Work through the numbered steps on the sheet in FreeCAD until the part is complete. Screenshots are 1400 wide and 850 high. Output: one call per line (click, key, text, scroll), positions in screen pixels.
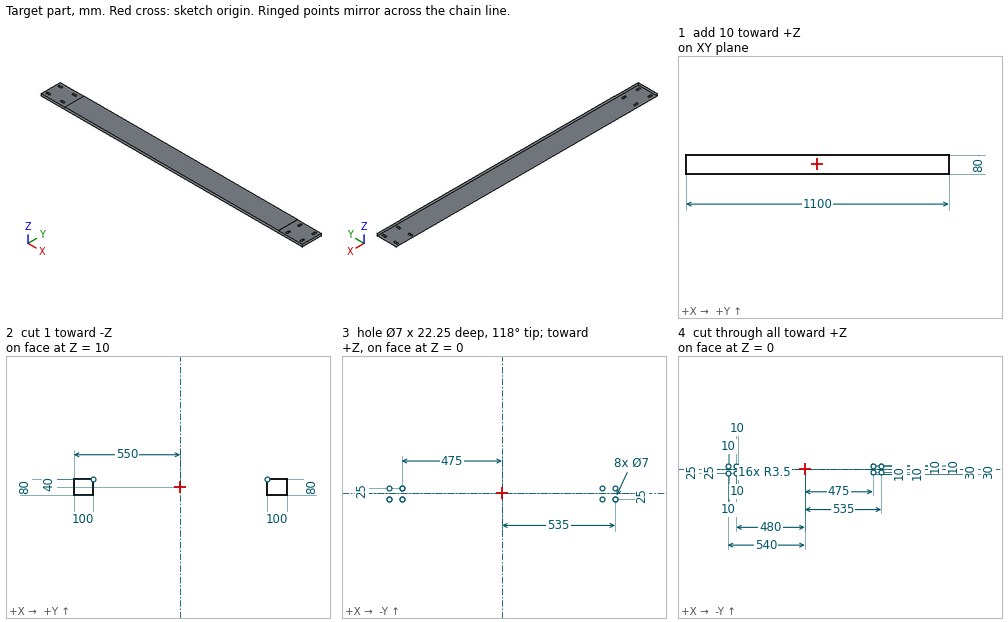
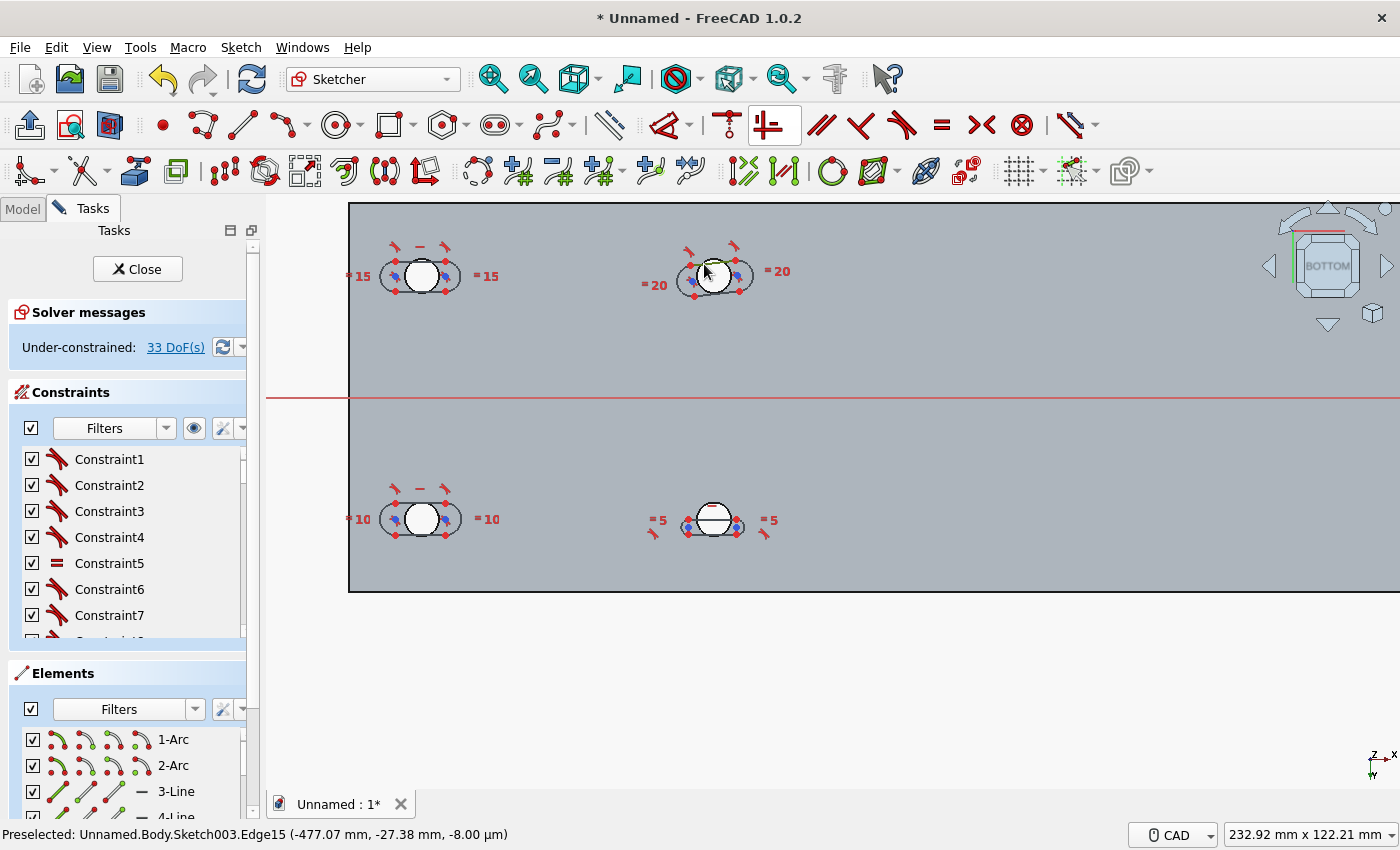
click(796, 126)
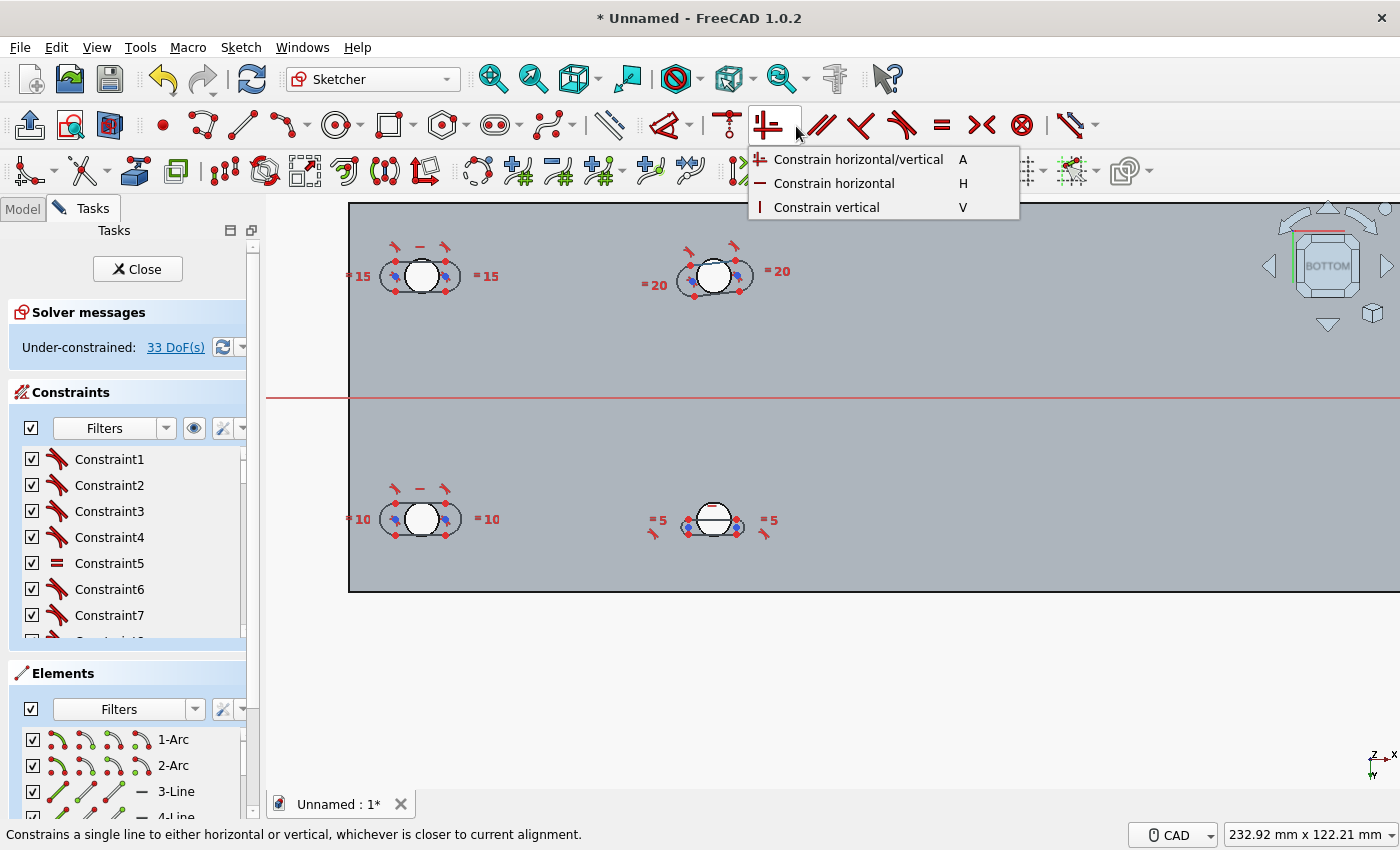
click(884, 183)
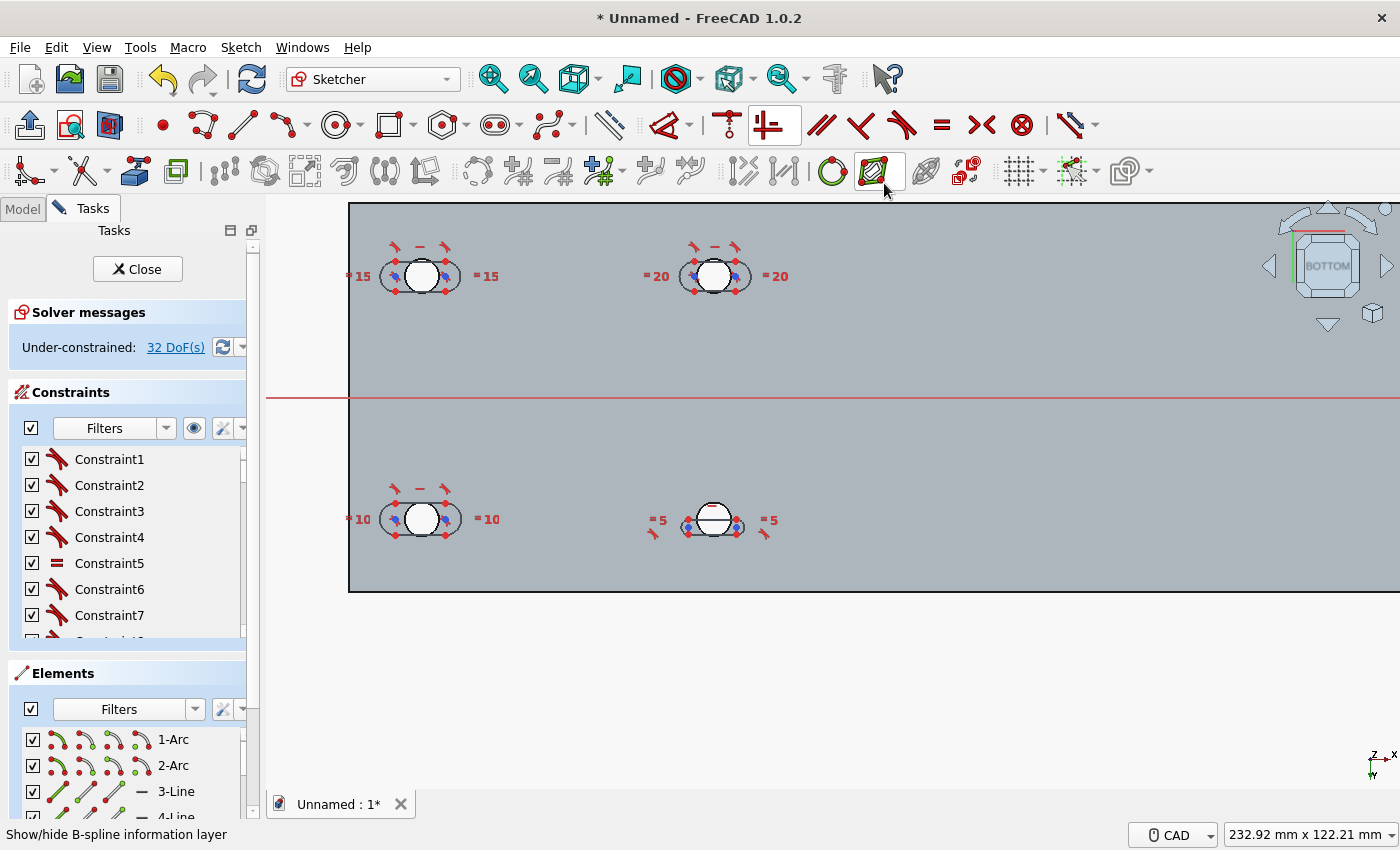
scroll(681, 527, up, 3)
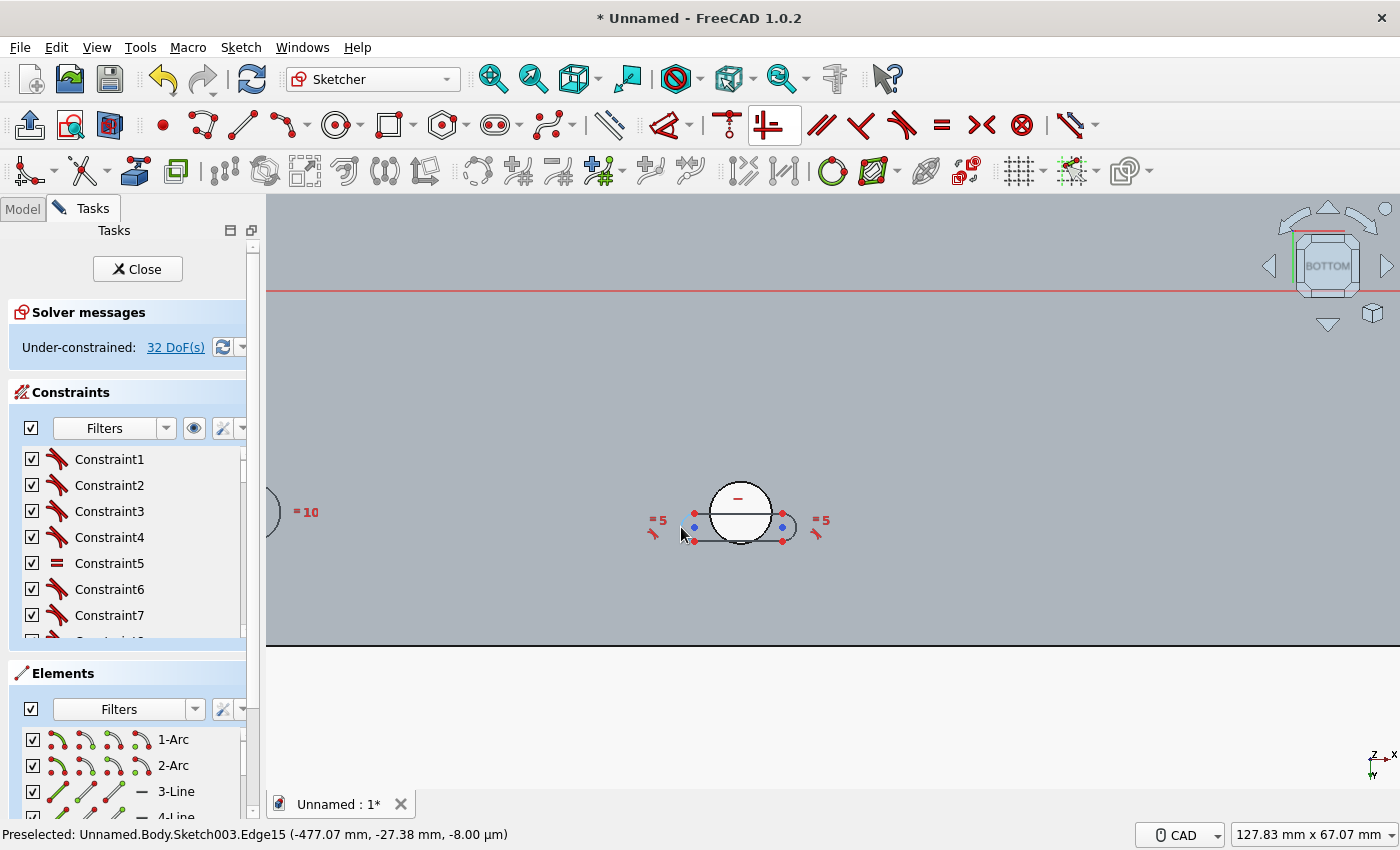
click(681, 527)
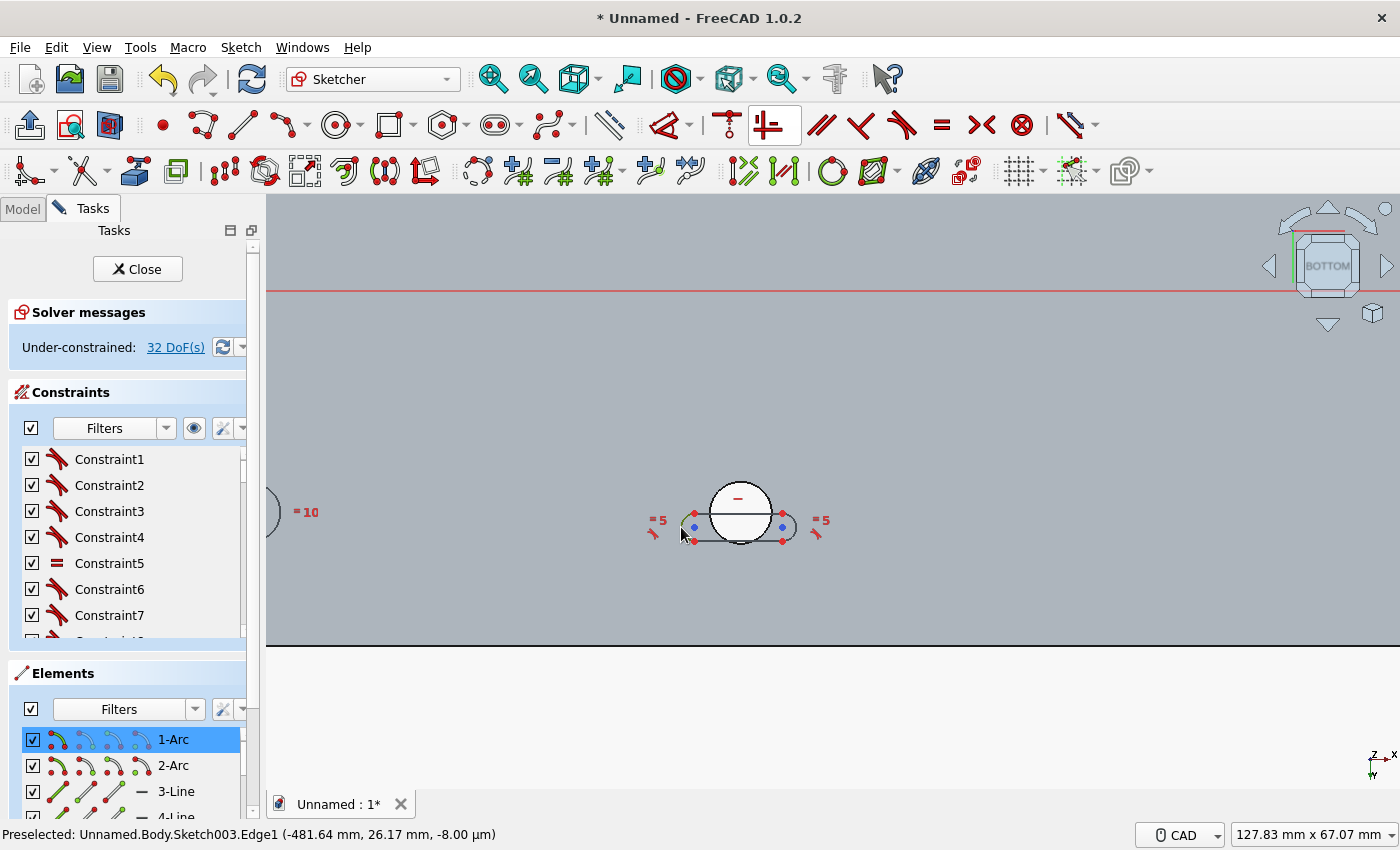
scroll(430, 508, down, 13)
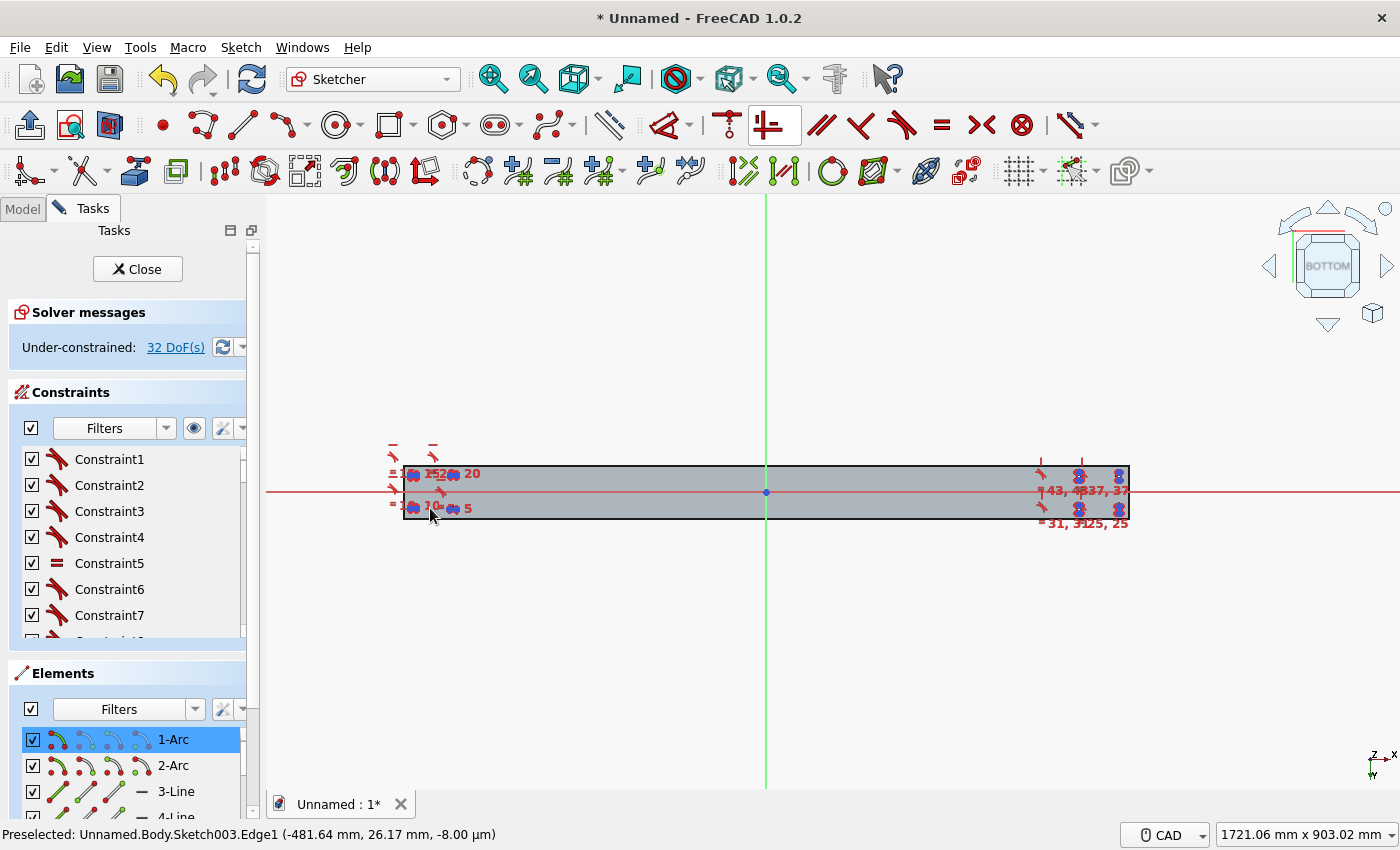
scroll(408, 508, up, 10)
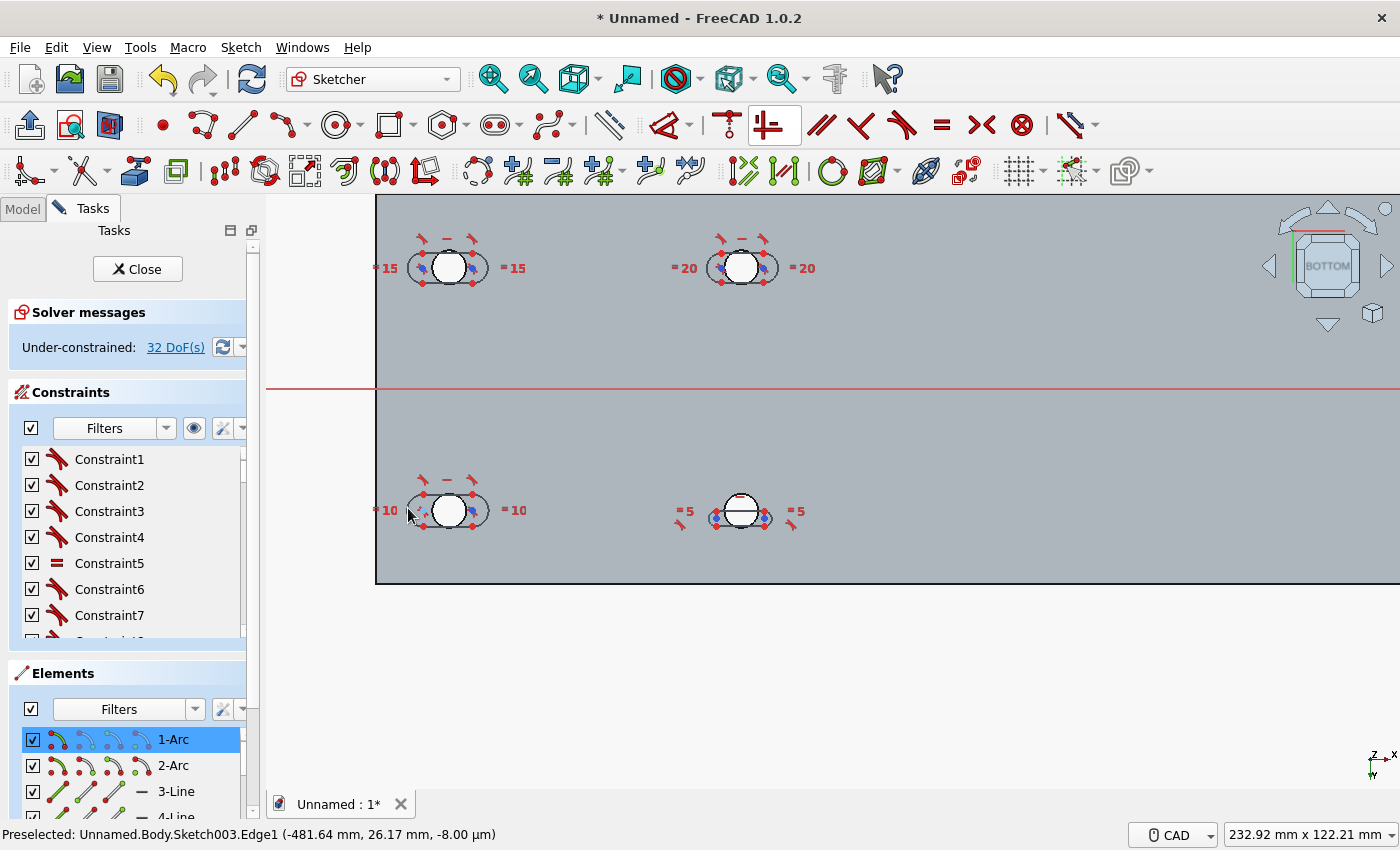
click(410, 501)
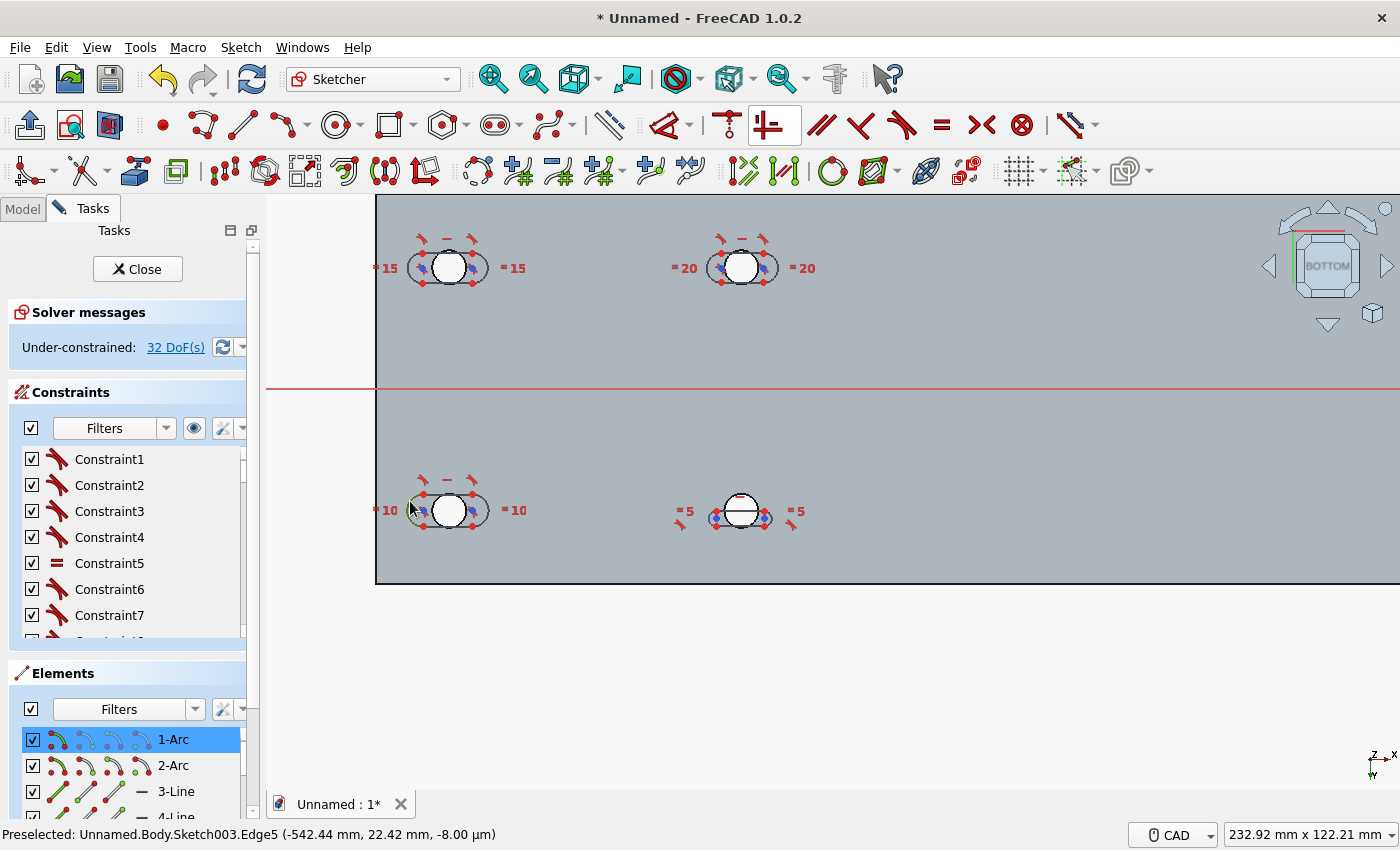
click(410, 259)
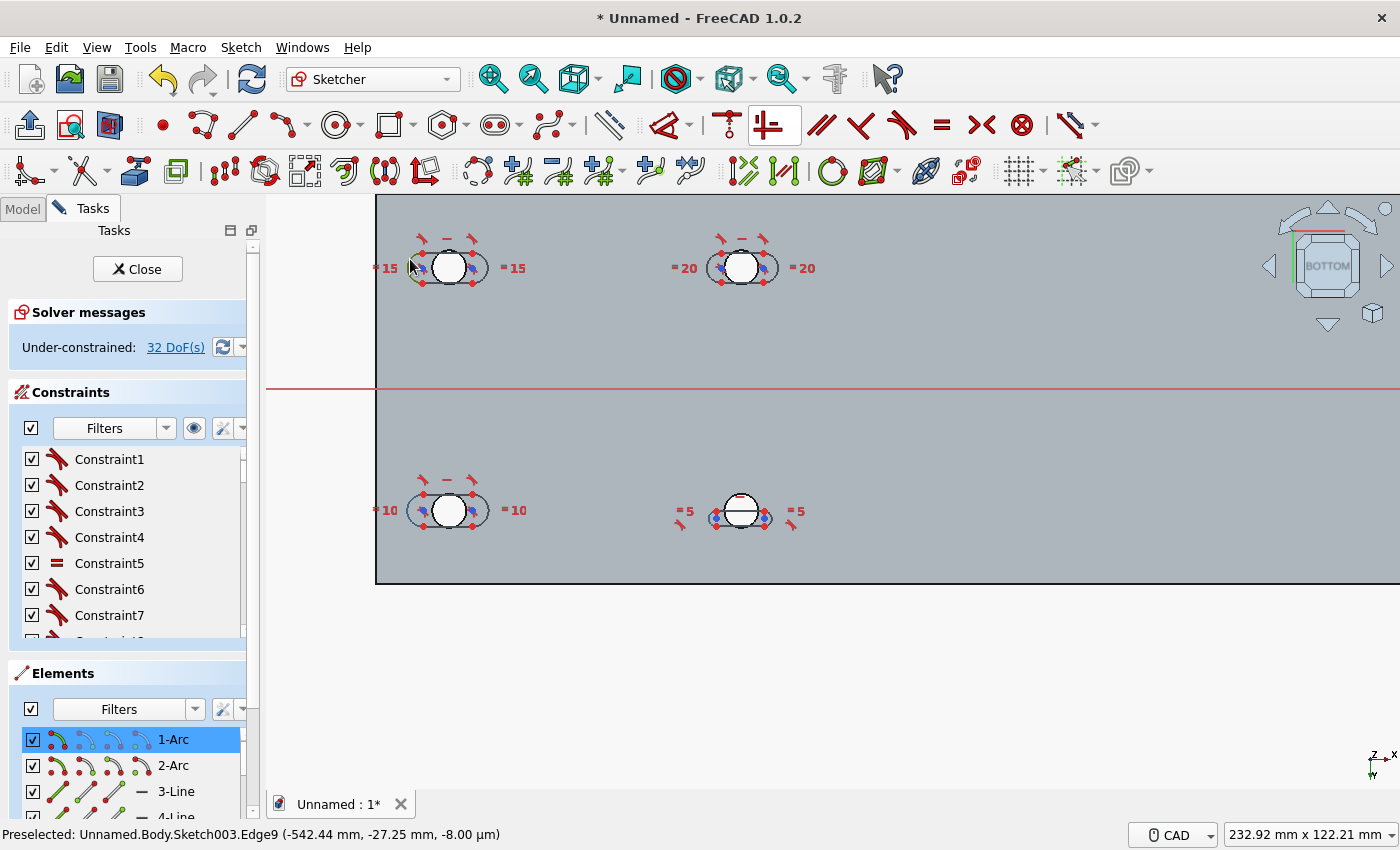
click(710, 259)